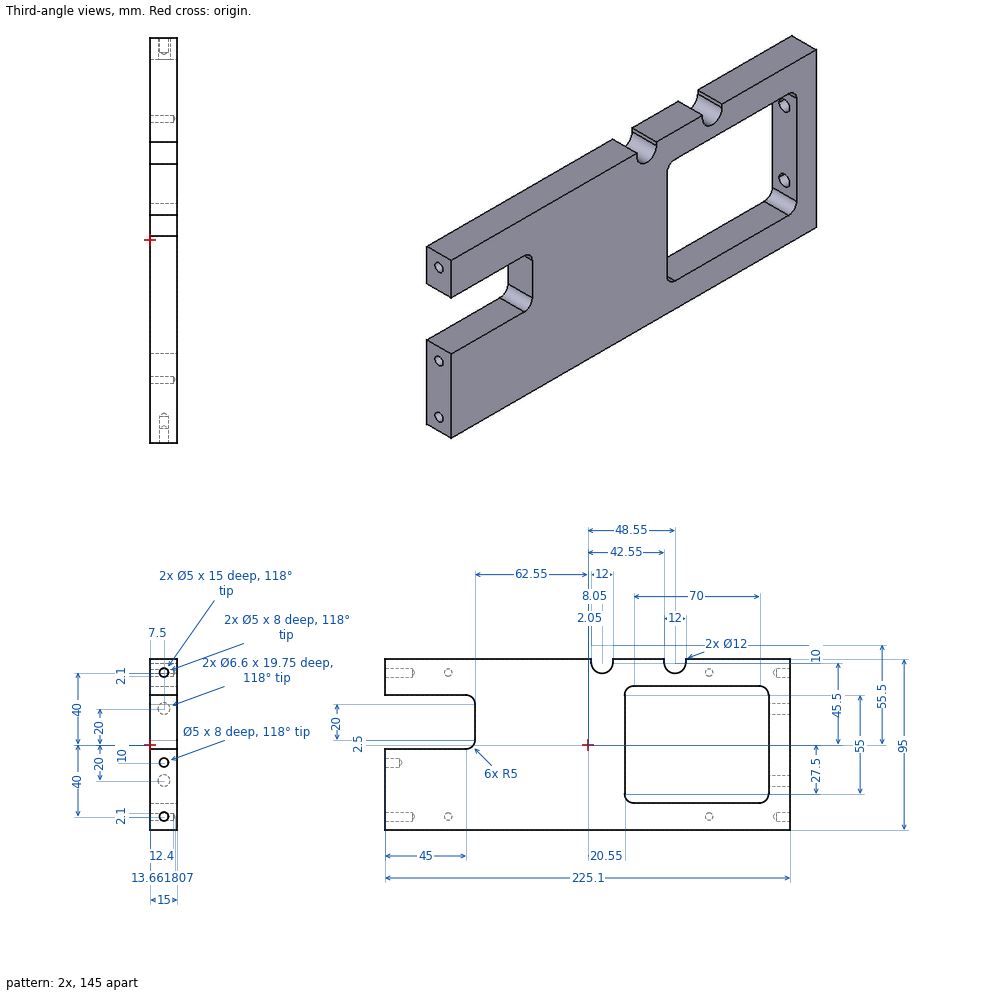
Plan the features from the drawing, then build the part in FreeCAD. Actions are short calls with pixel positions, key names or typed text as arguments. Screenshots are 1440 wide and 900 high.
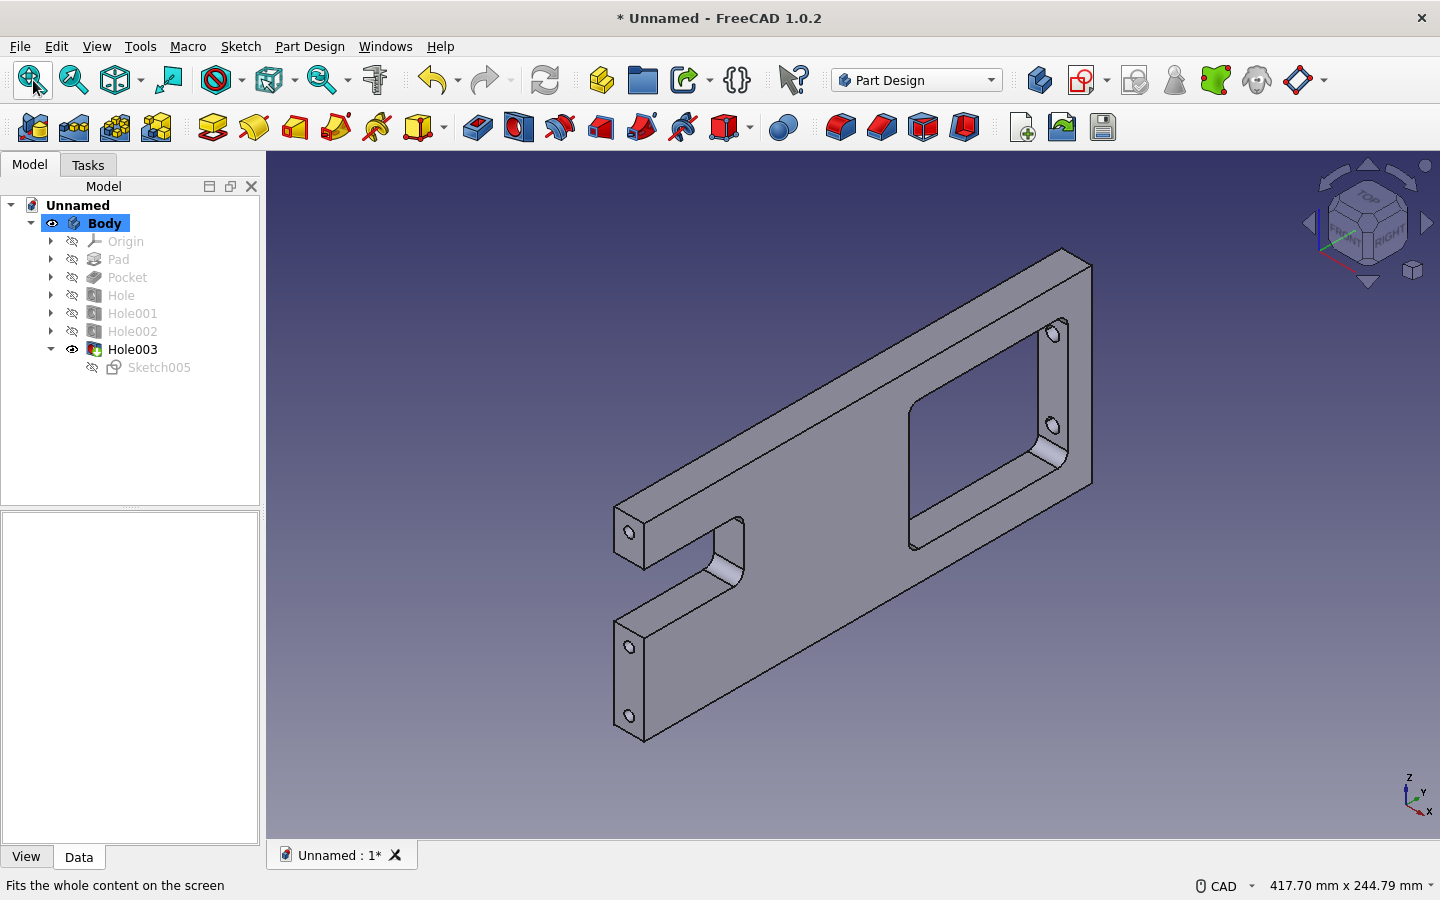
click(804, 571)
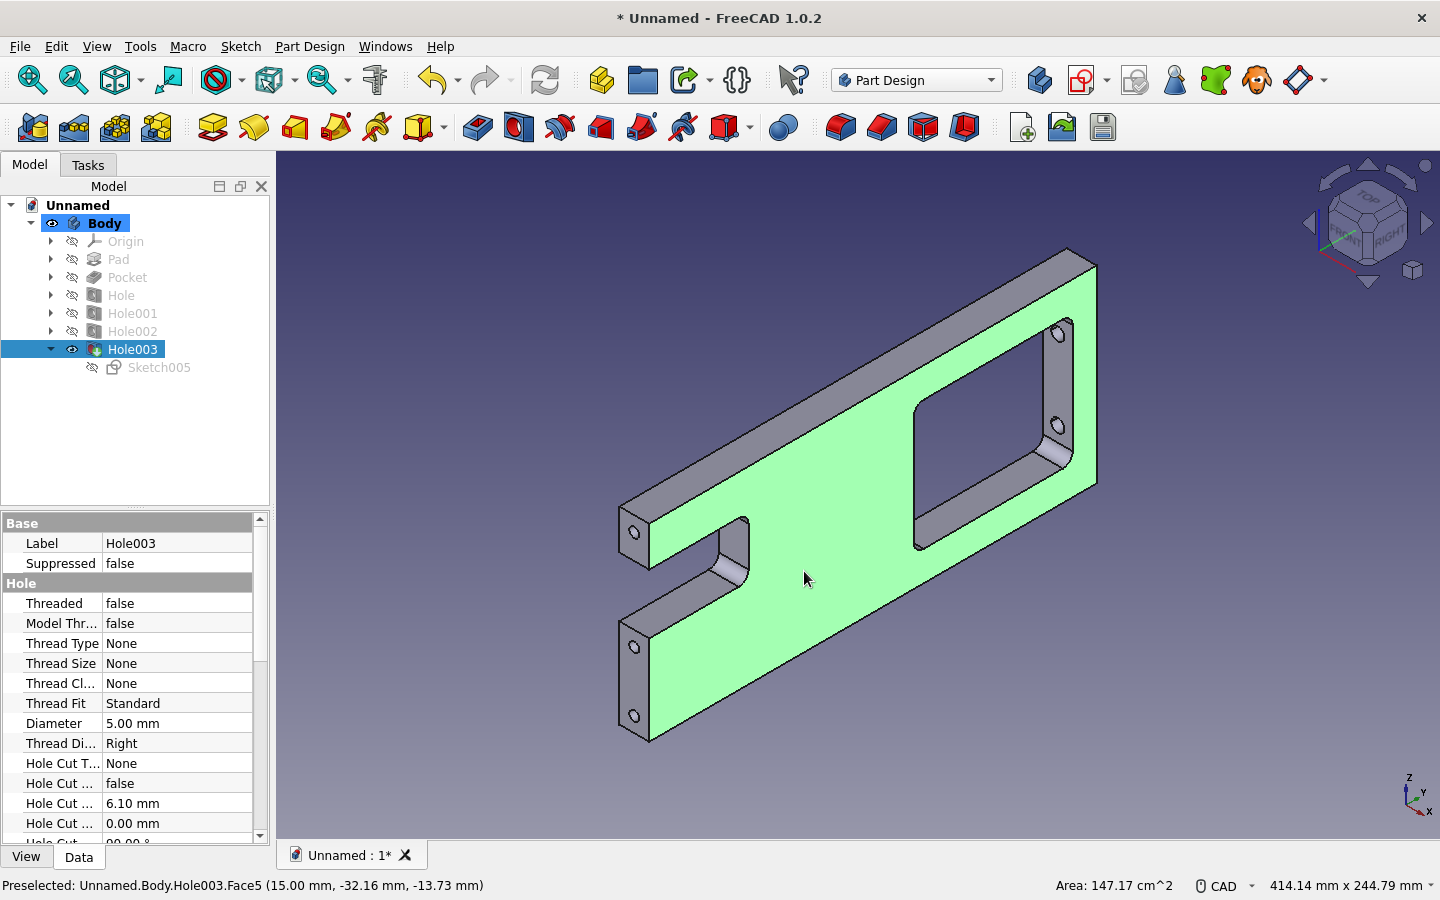
click(1080, 80)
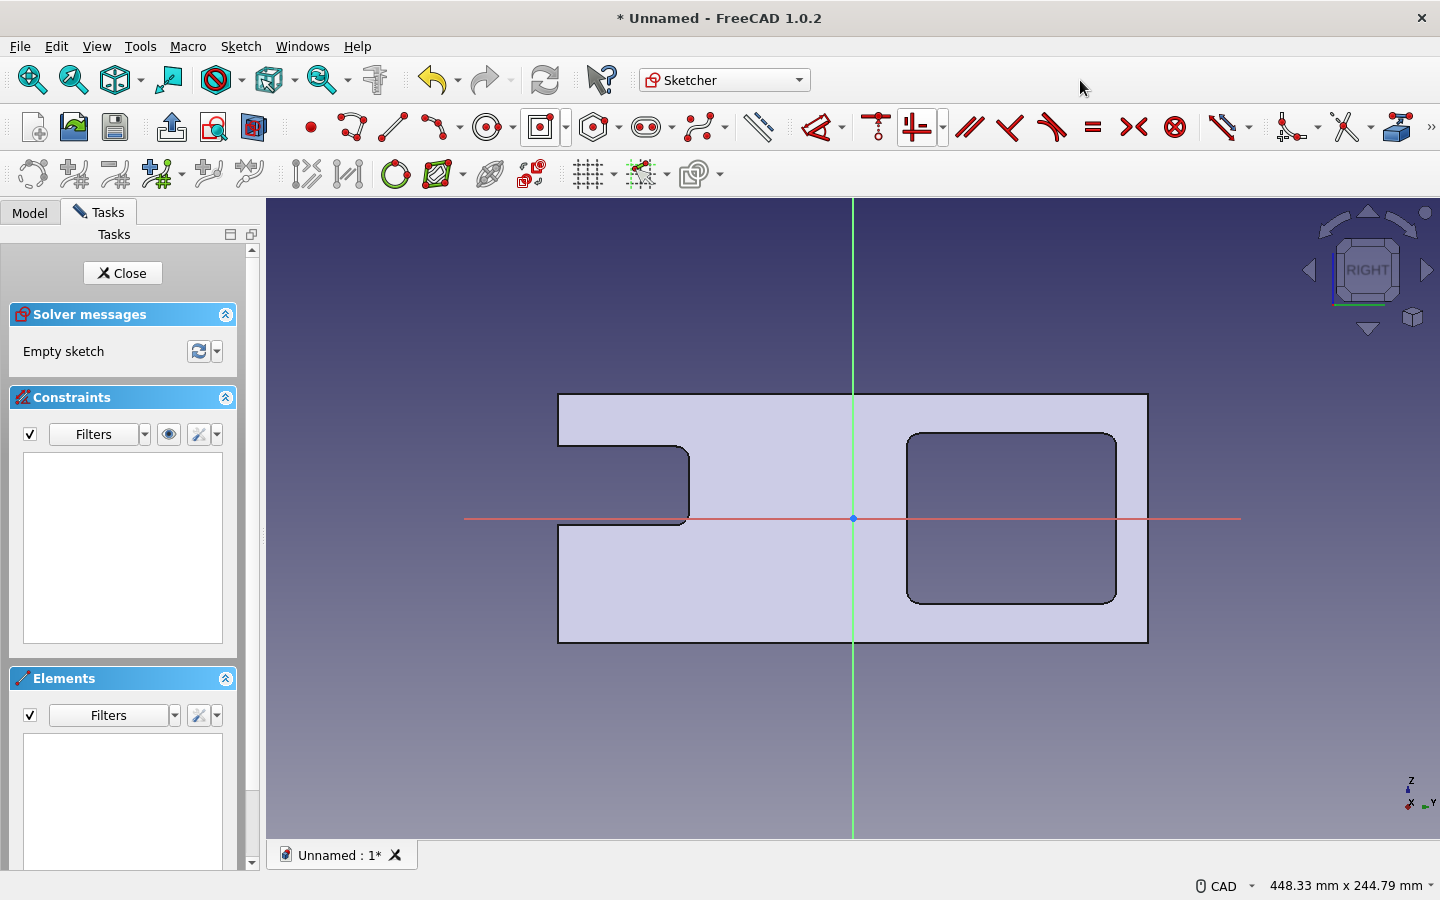
scroll(985, 422, up, 6)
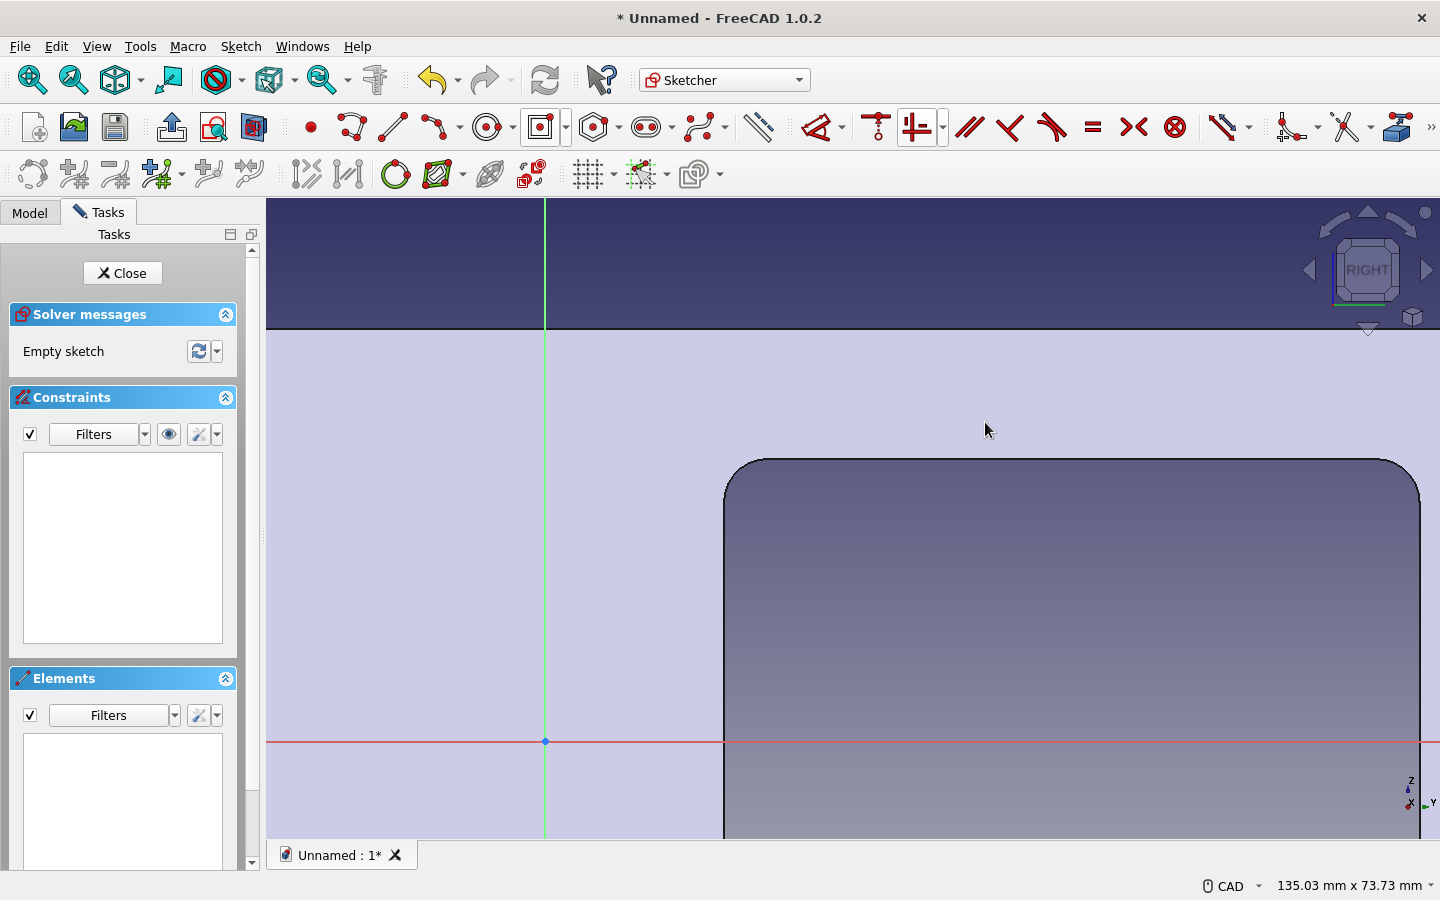
click(486, 128)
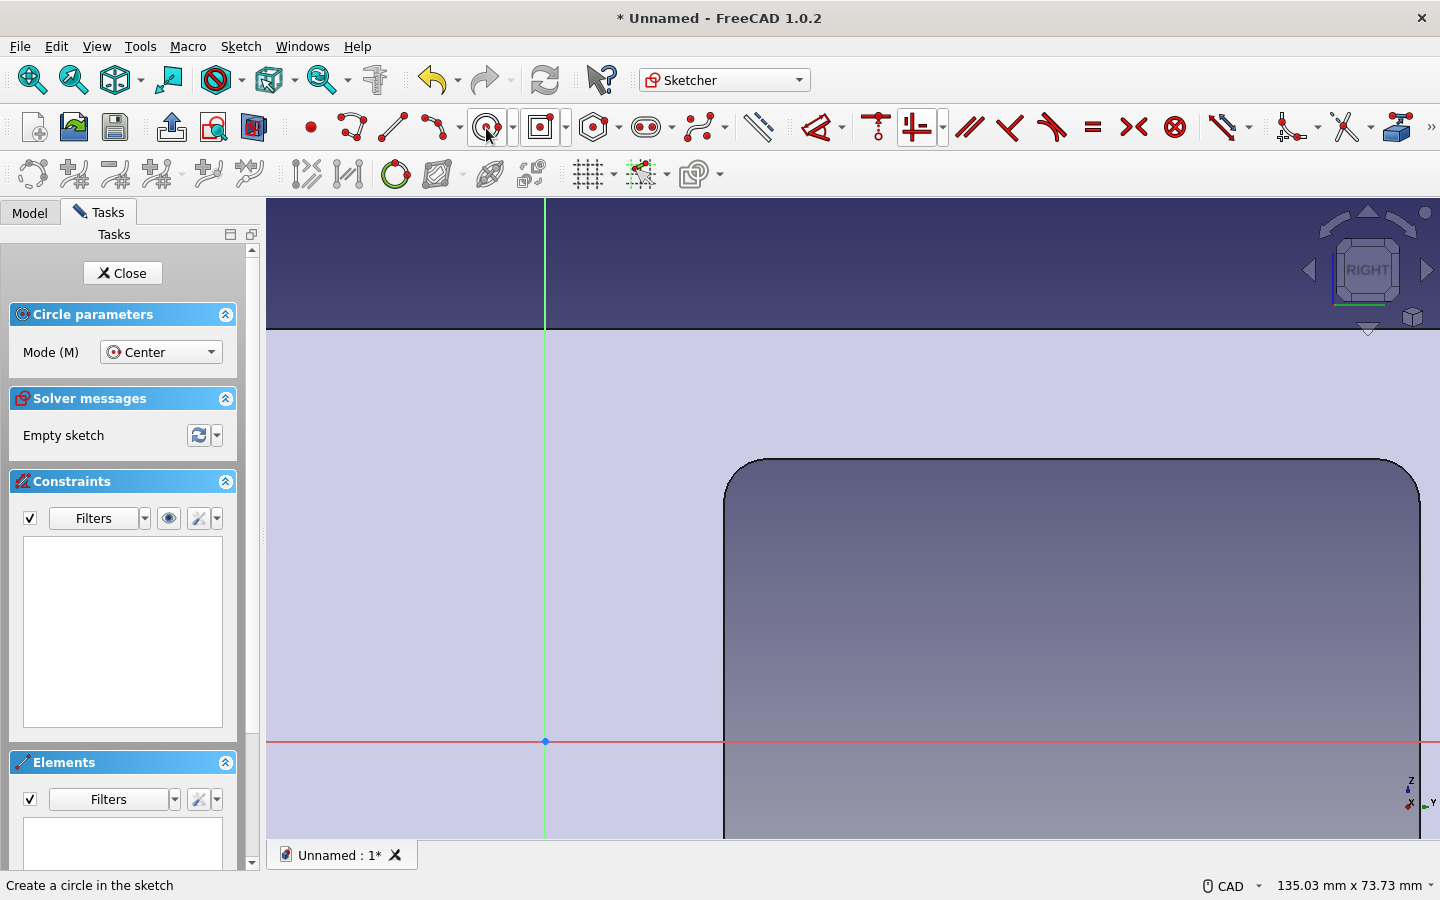
click(967, 346)
move(1004, 309)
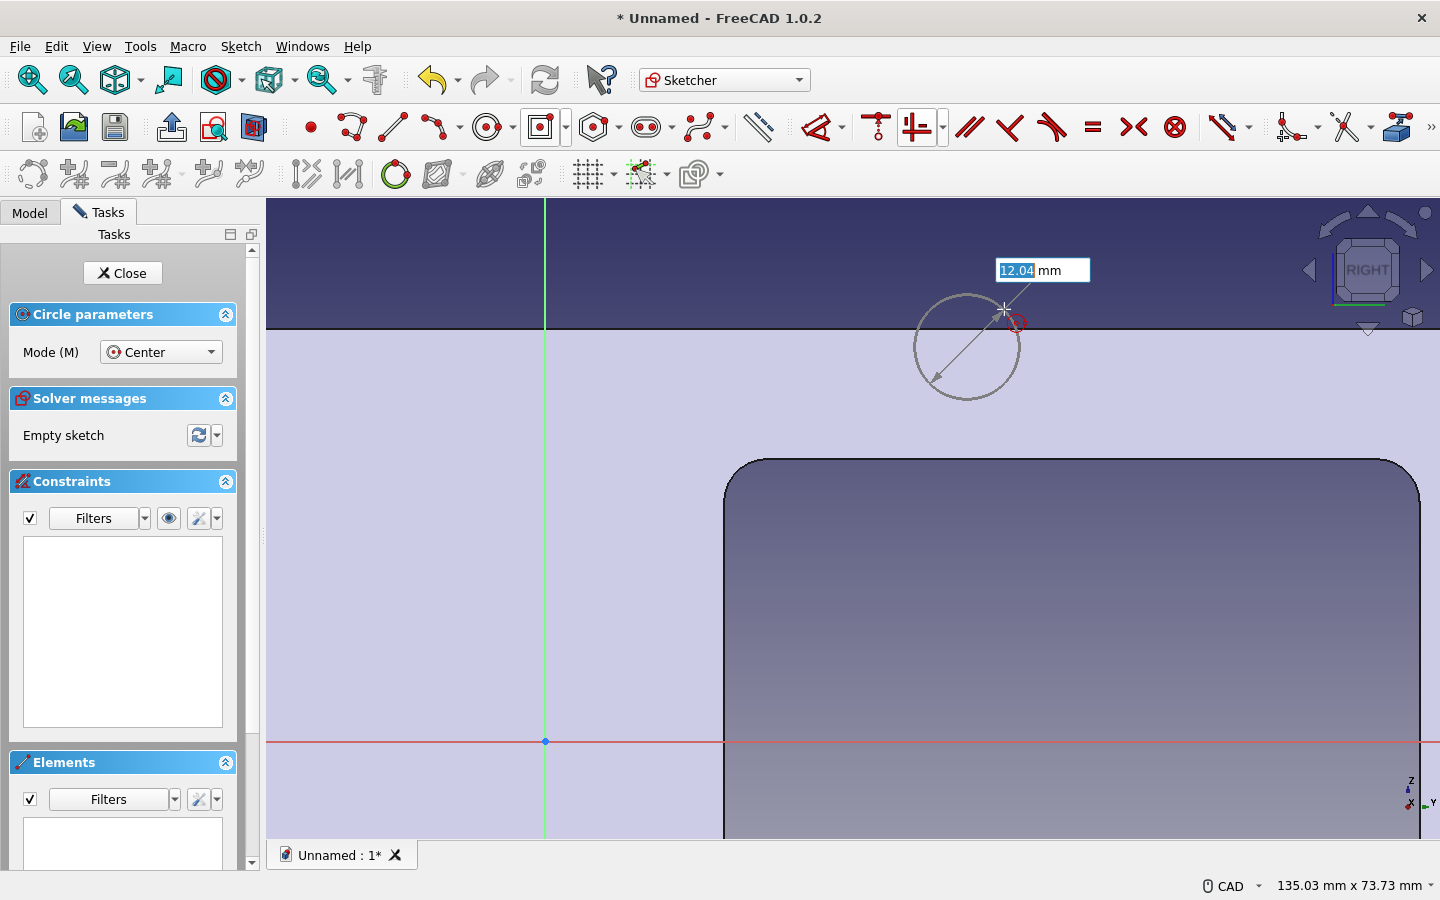
text(12)
key(Return)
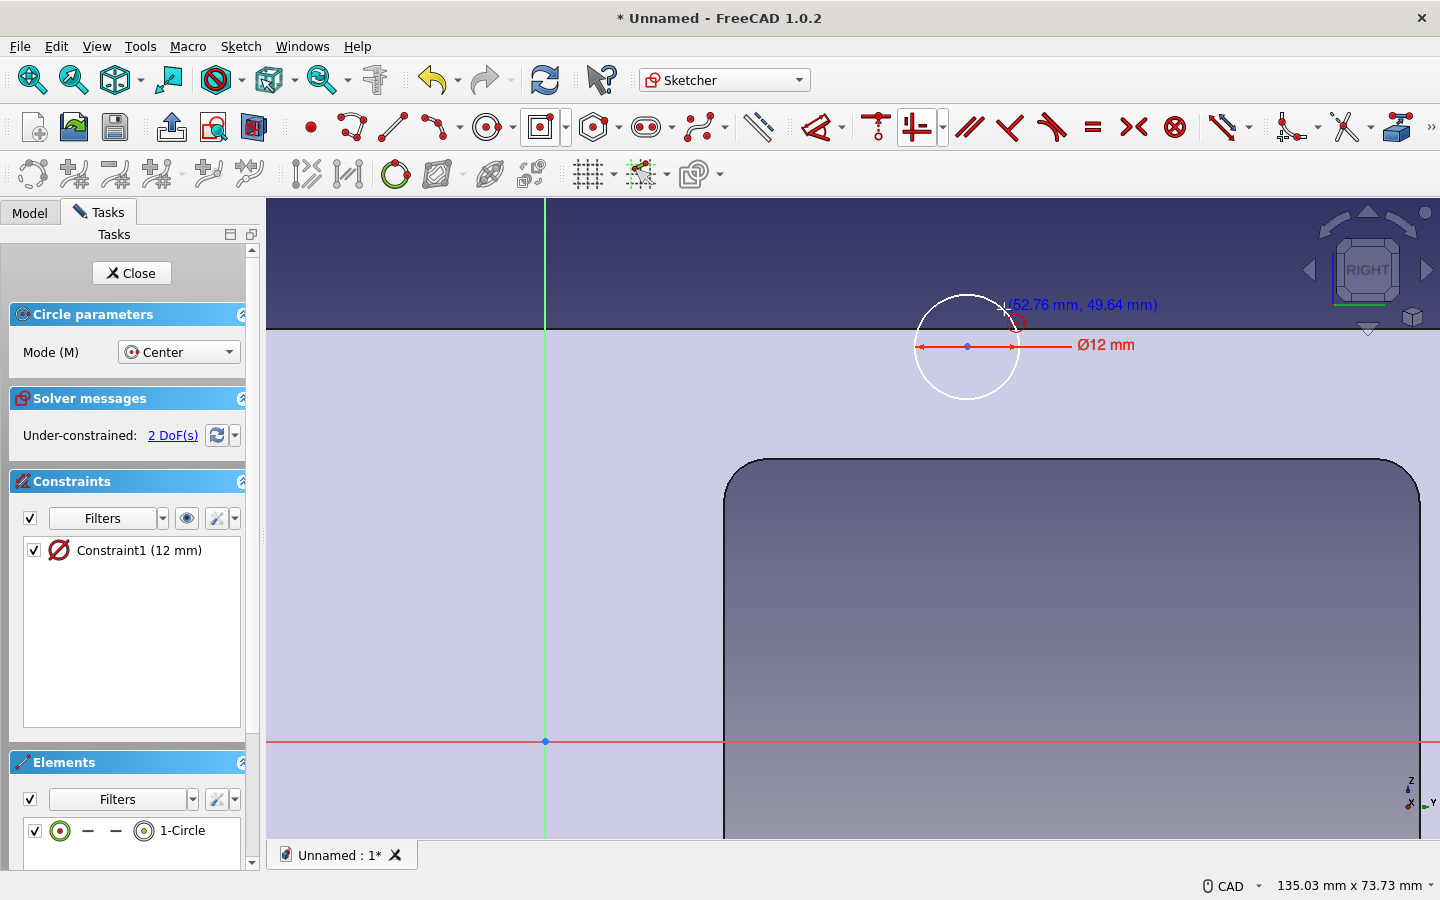
click(615, 346)
move(652, 309)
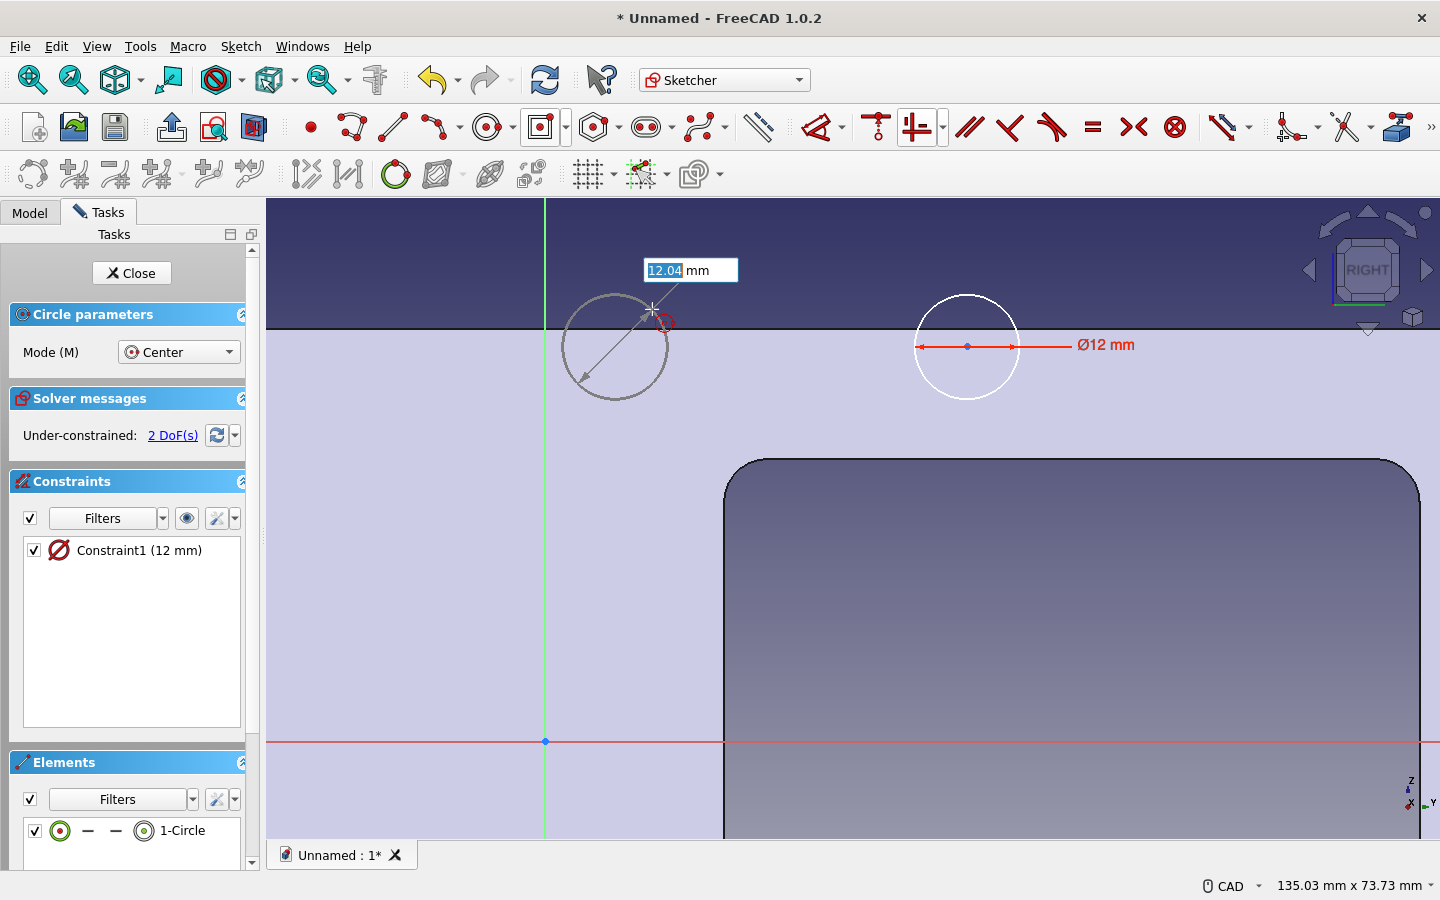
text(12)
key(Return)
key(Escape)